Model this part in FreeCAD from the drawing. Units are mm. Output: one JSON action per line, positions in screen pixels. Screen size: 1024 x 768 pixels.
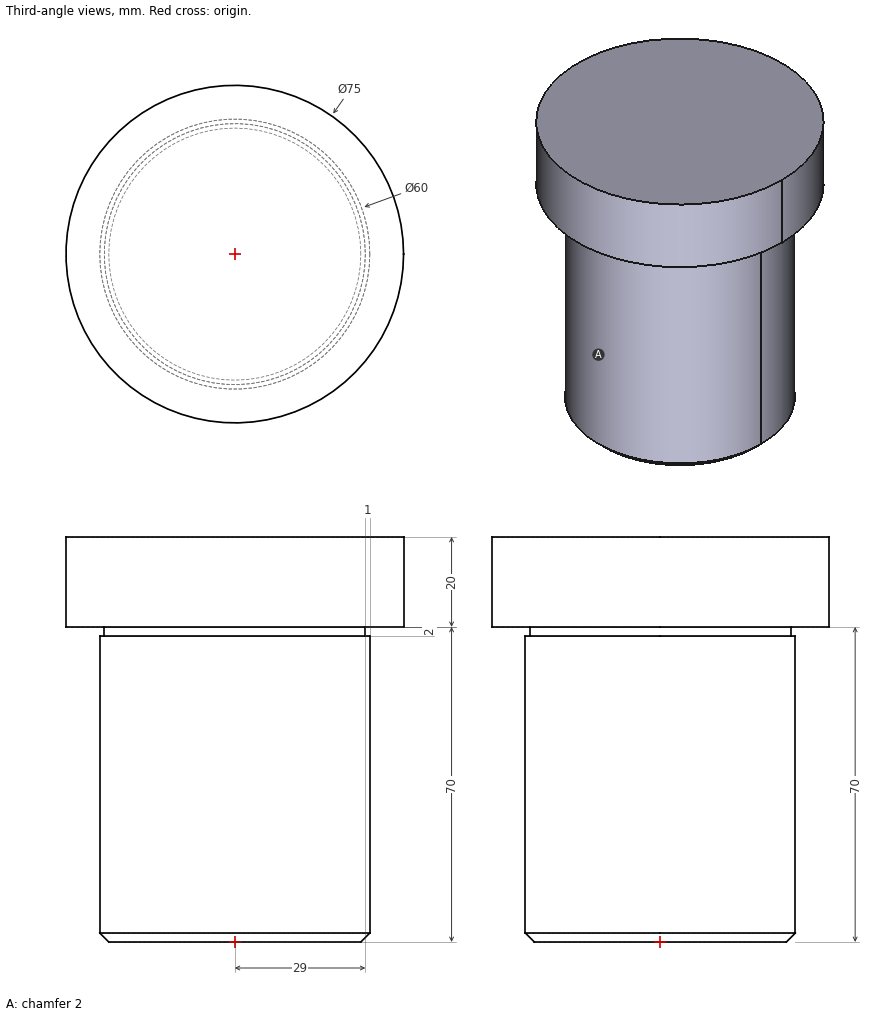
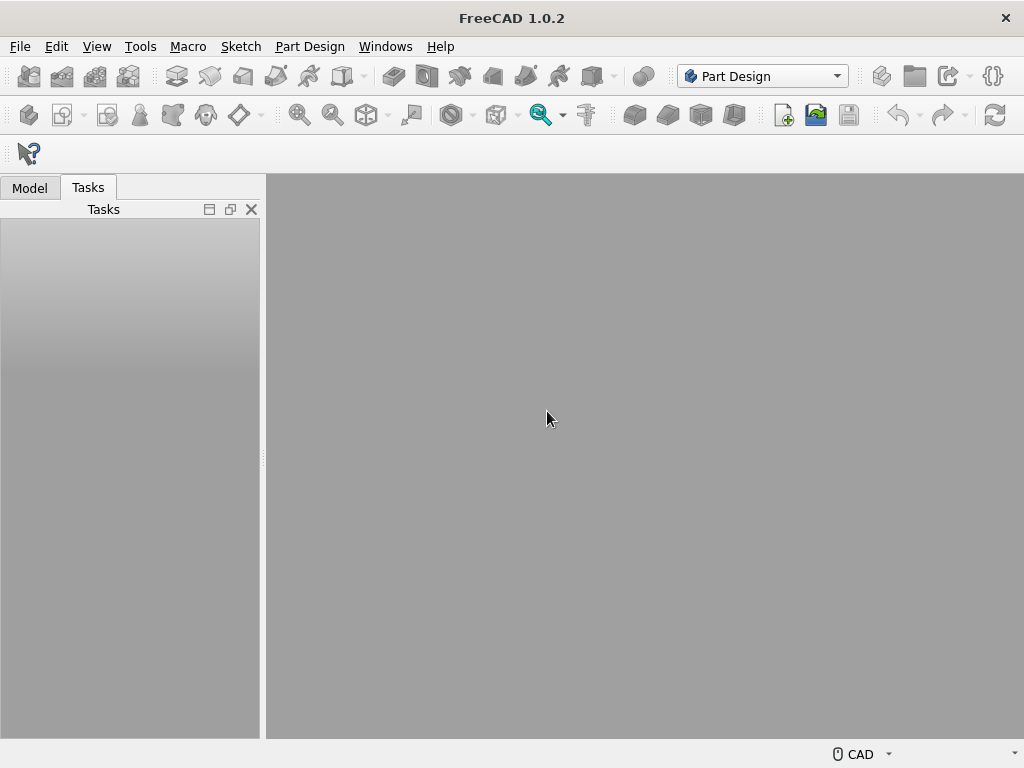
{"action": "key", "text": "ctrl+n"}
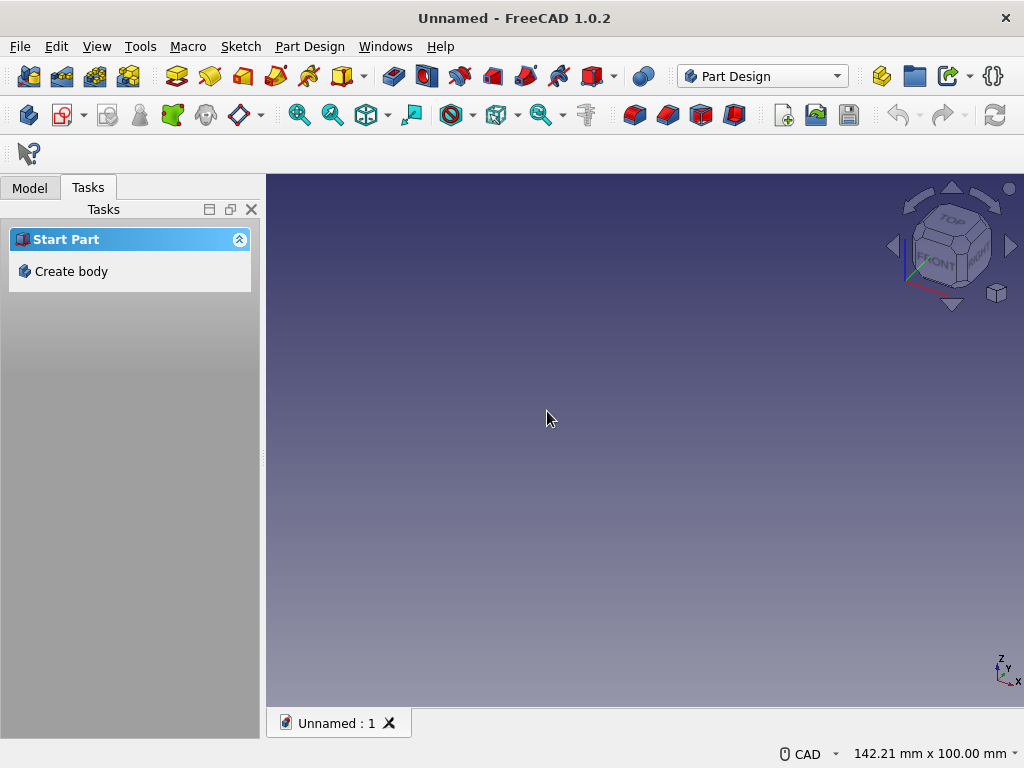
{"action": "left_click", "coordinate": [62, 116]}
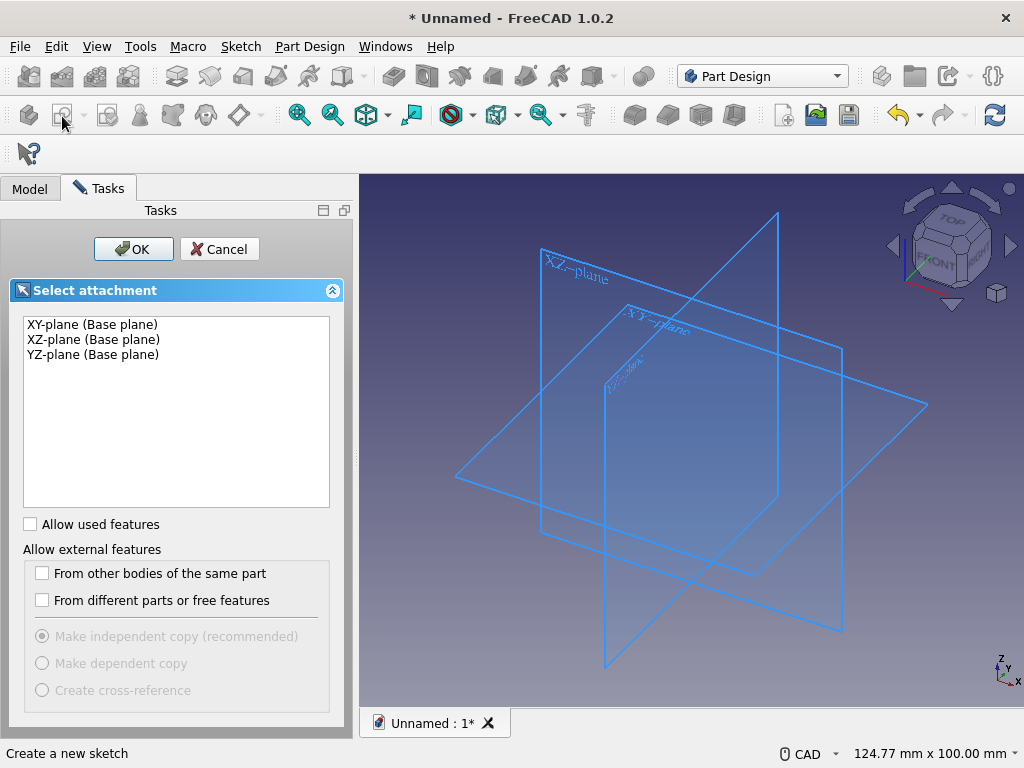
{"action": "left_click", "coordinate": [84, 324]}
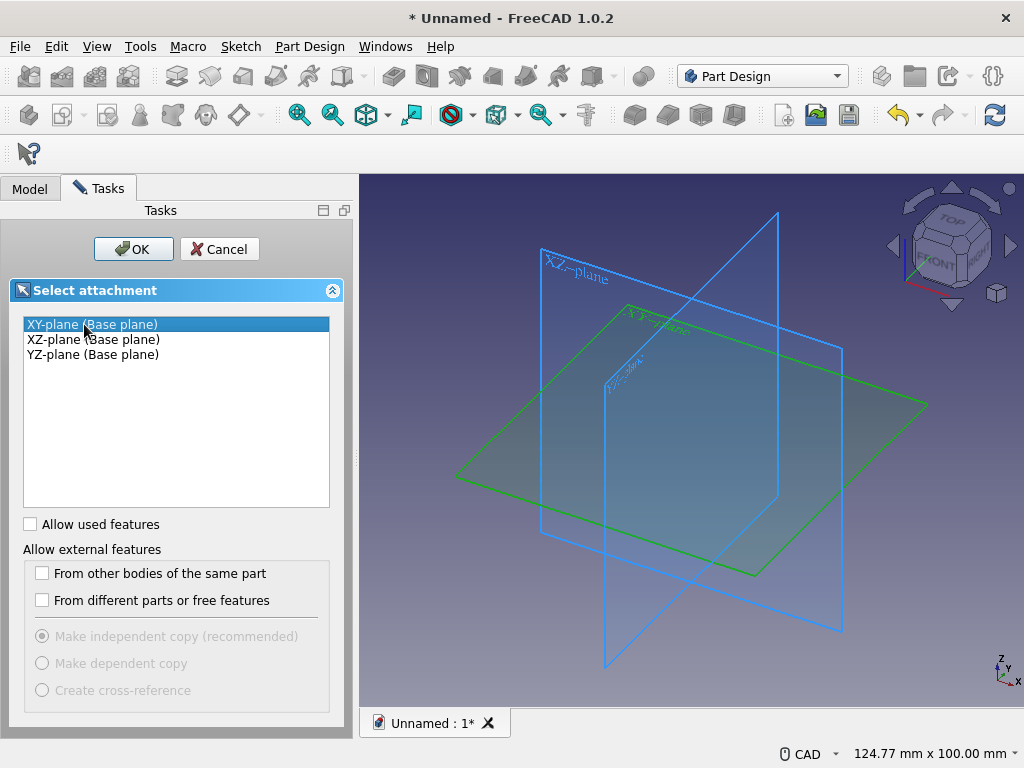
{"action": "left_click", "coordinate": [134, 249]}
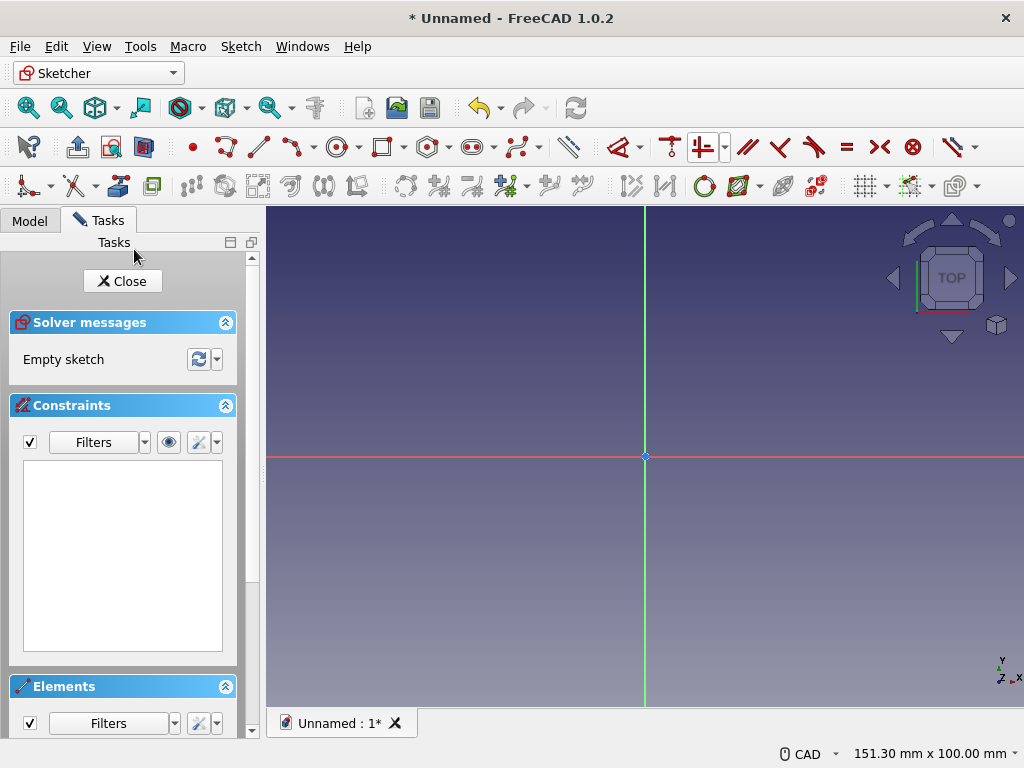
{"action": "key", "text": "g c"}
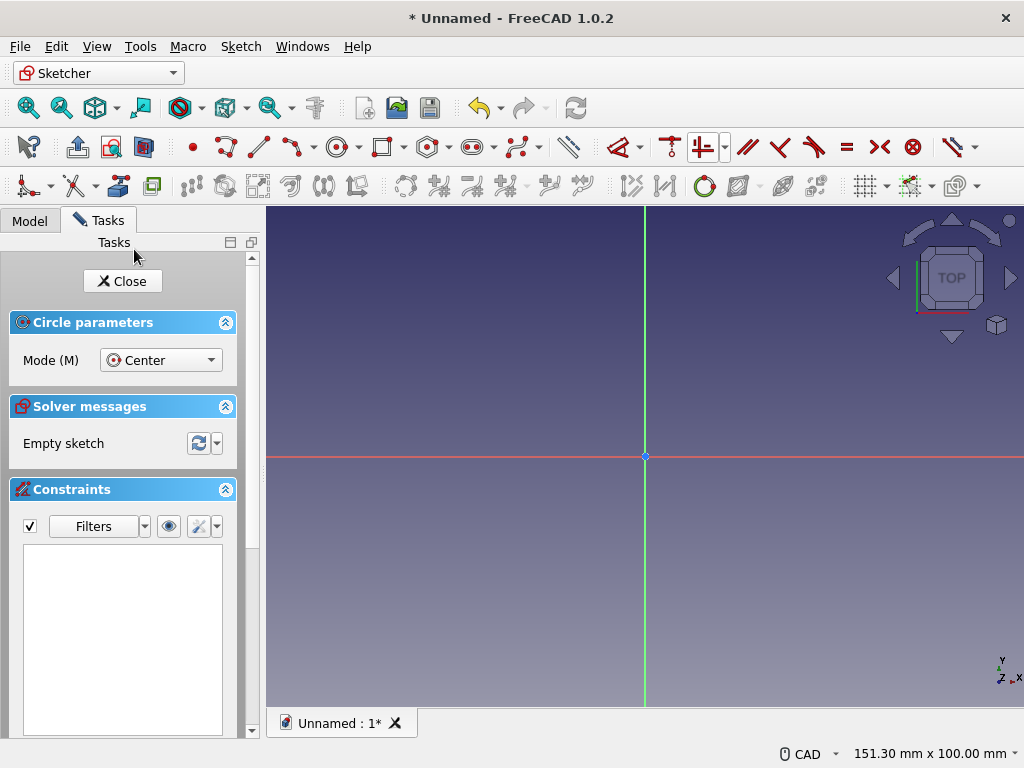
{"action": "left_click", "coordinate": [645, 456]}
{"action": "mouse_move", "coordinate": [751, 350]}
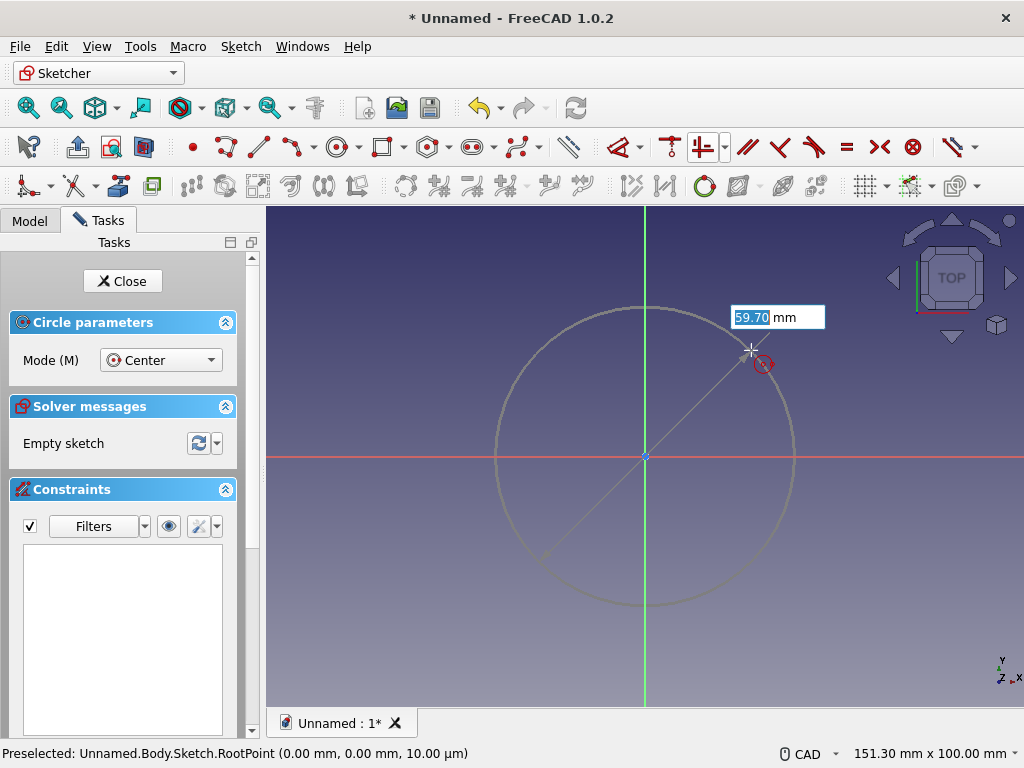
{"action": "type", "text": "60"}
{"action": "key", "text": "Return"}
{"action": "key", "text": "Escape"}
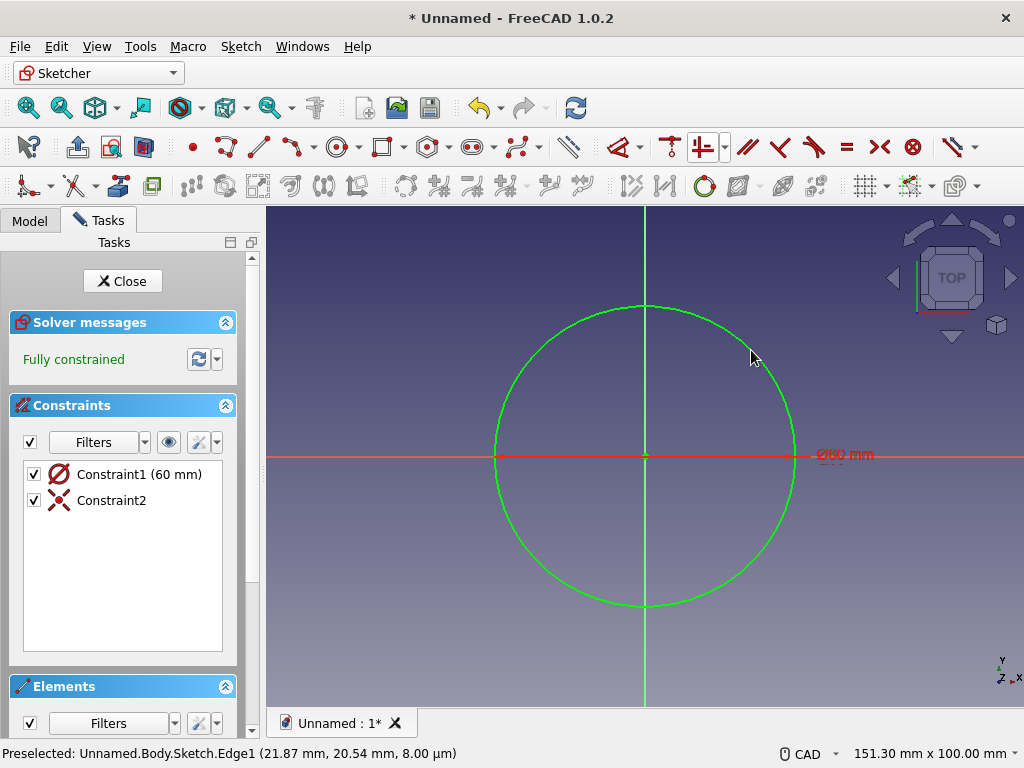
{"action": "left_click", "coordinate": [123, 281]}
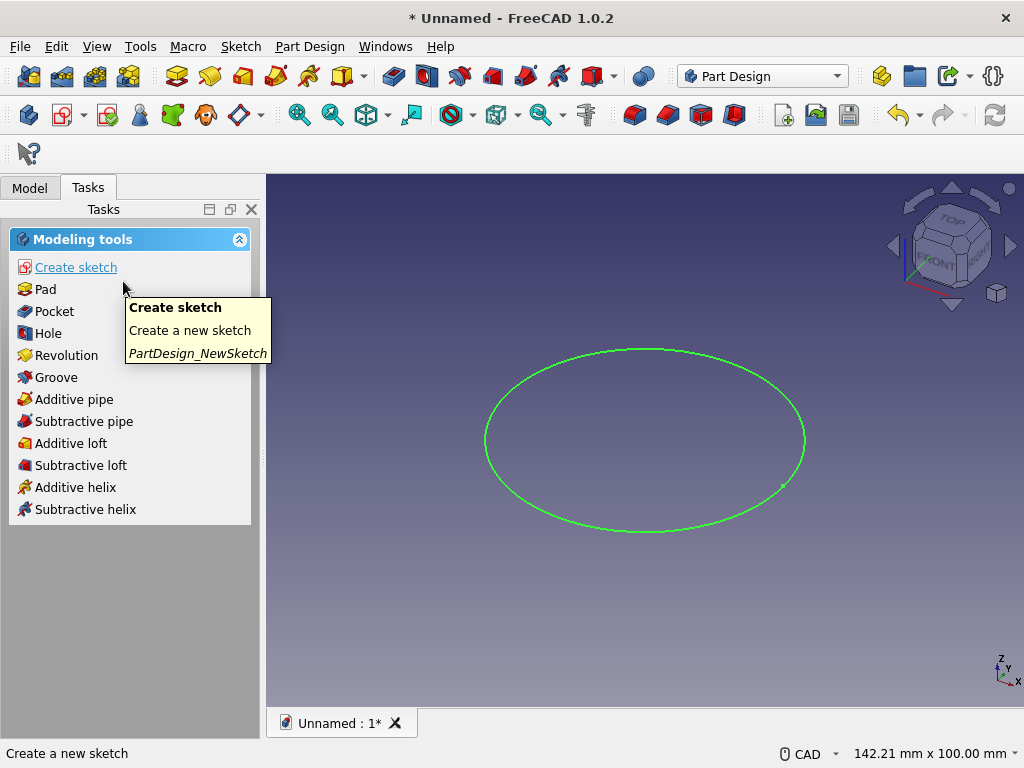
{"action": "left_click", "coordinate": [177, 76]}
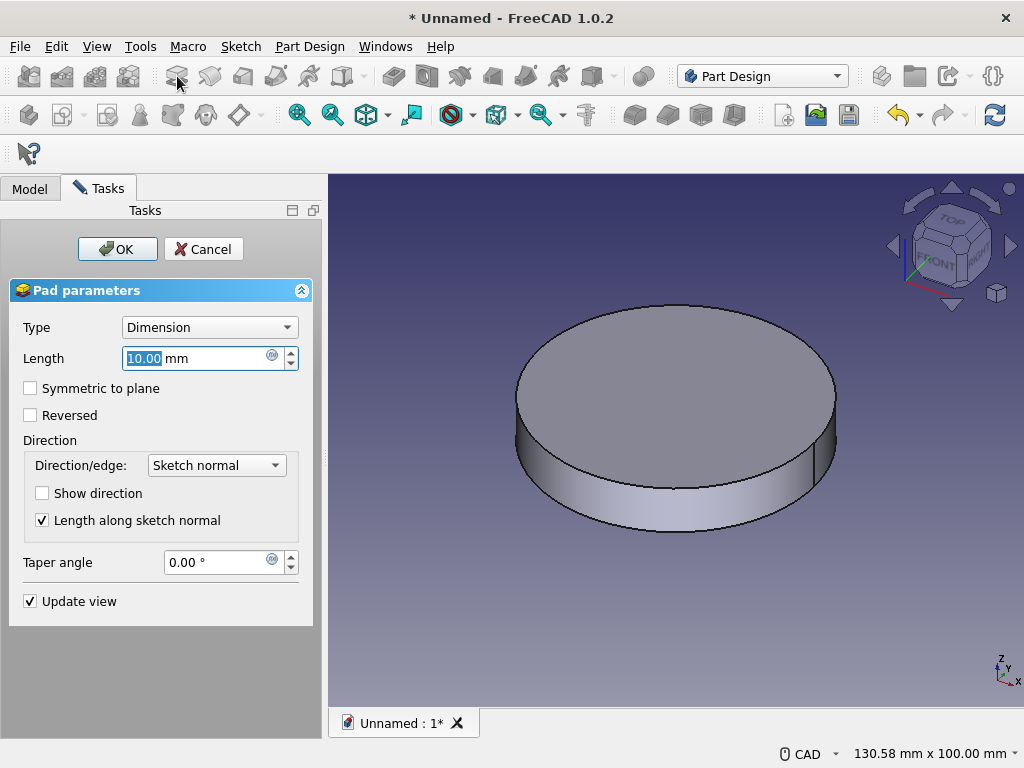
{"action": "type", "text": "70"}
{"action": "key", "text": "Tab"}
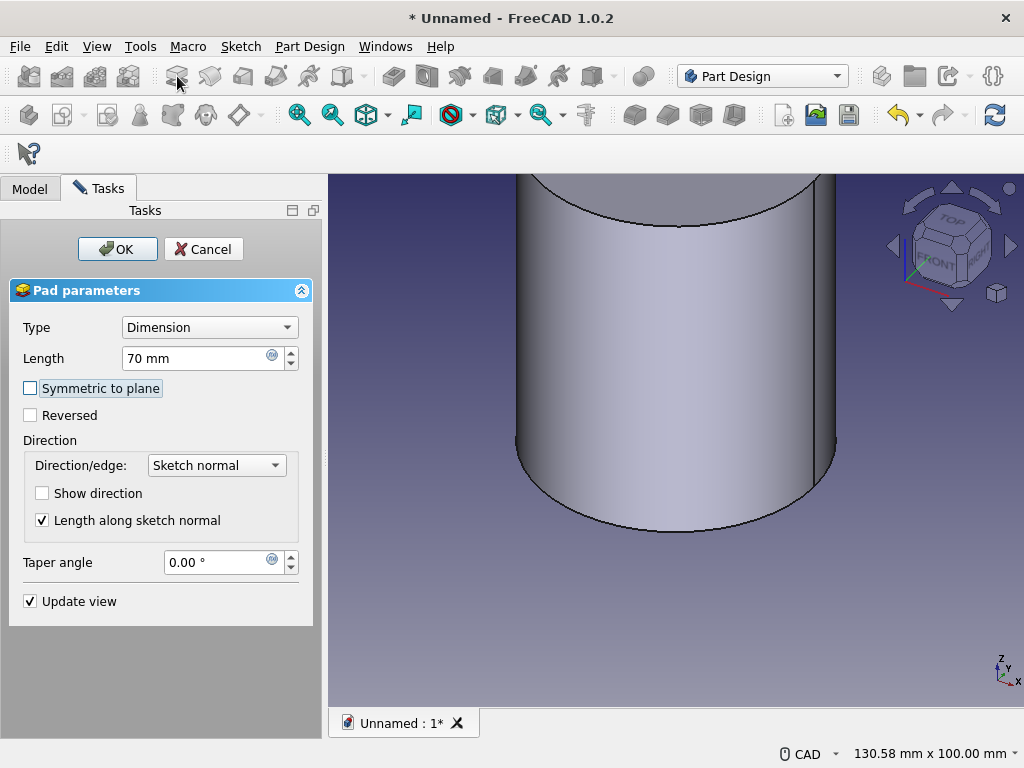
{"action": "left_click", "coordinate": [118, 249]}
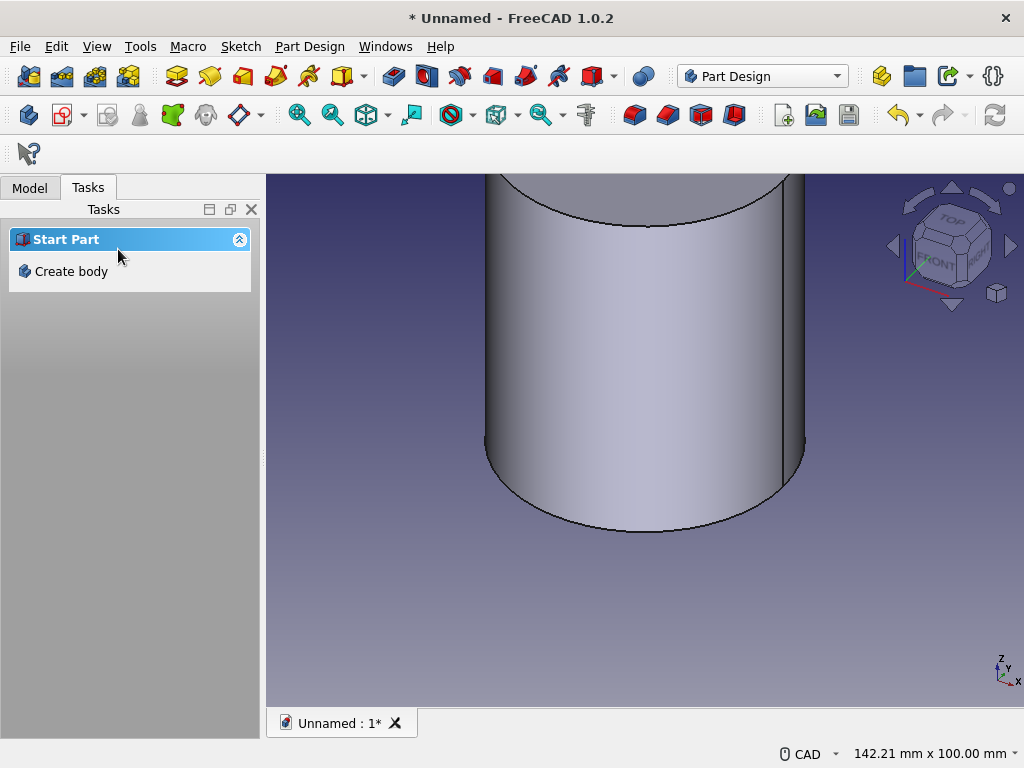
{"action": "key", "text": "v f"}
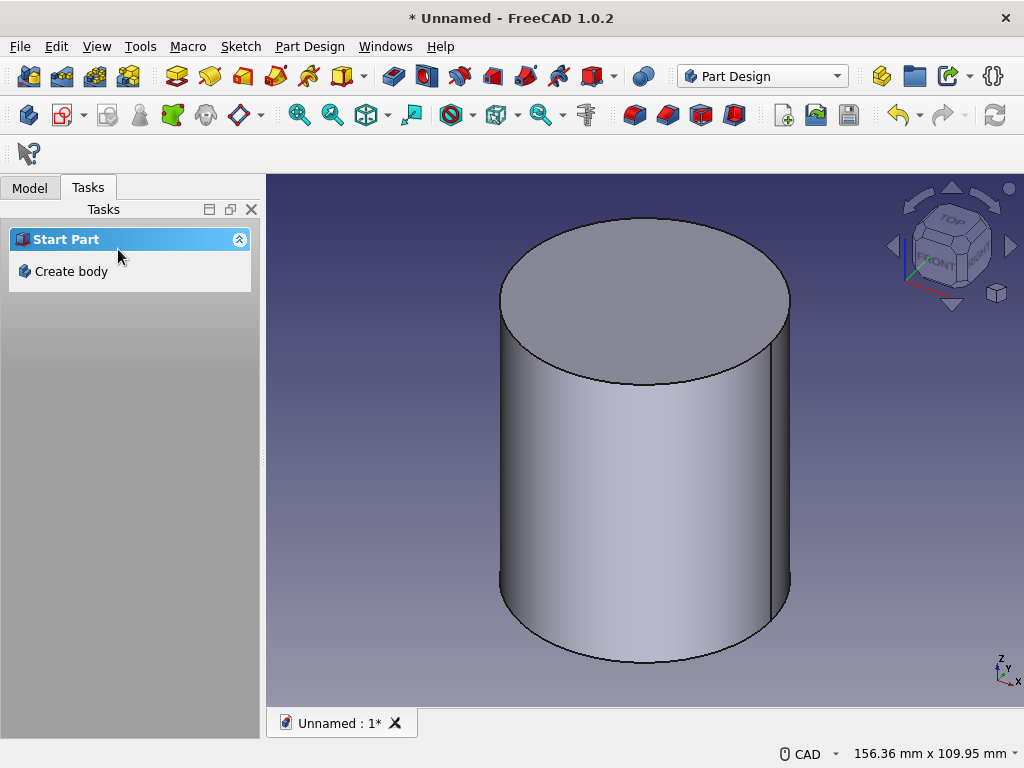
{"action": "left_click", "coordinate": [645, 300]}